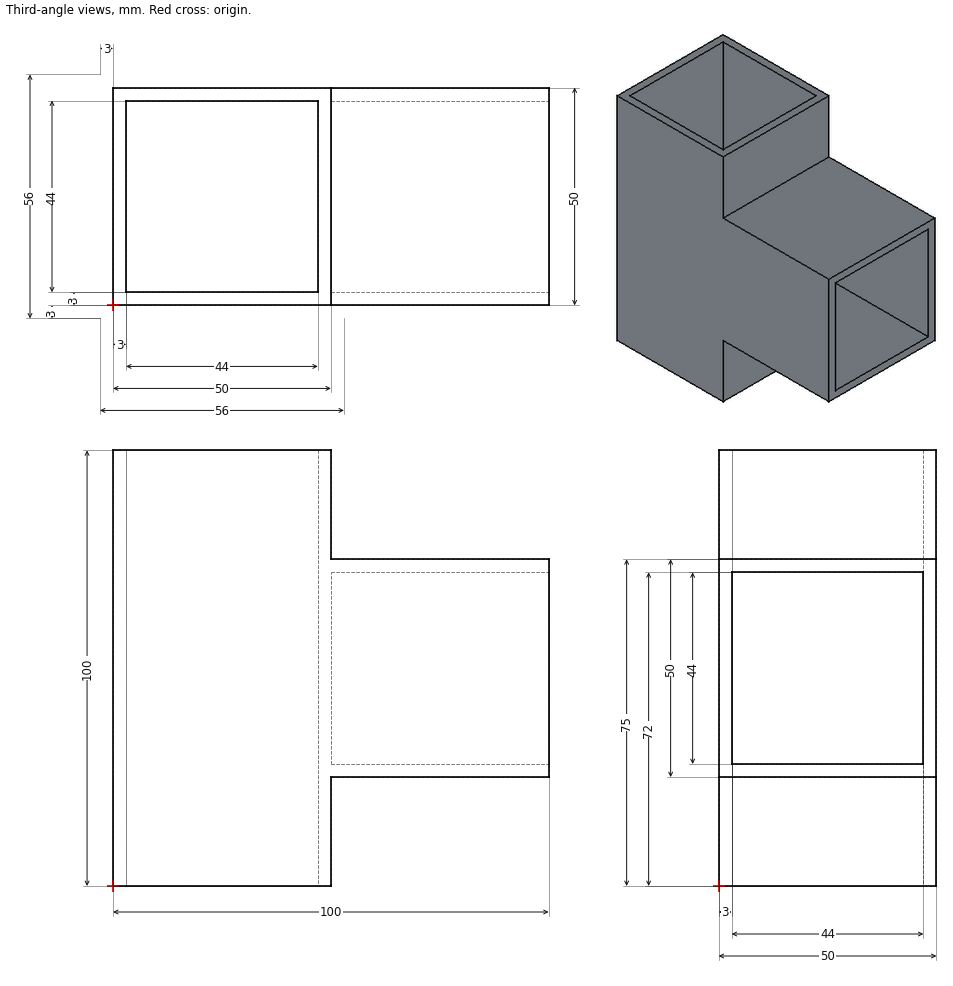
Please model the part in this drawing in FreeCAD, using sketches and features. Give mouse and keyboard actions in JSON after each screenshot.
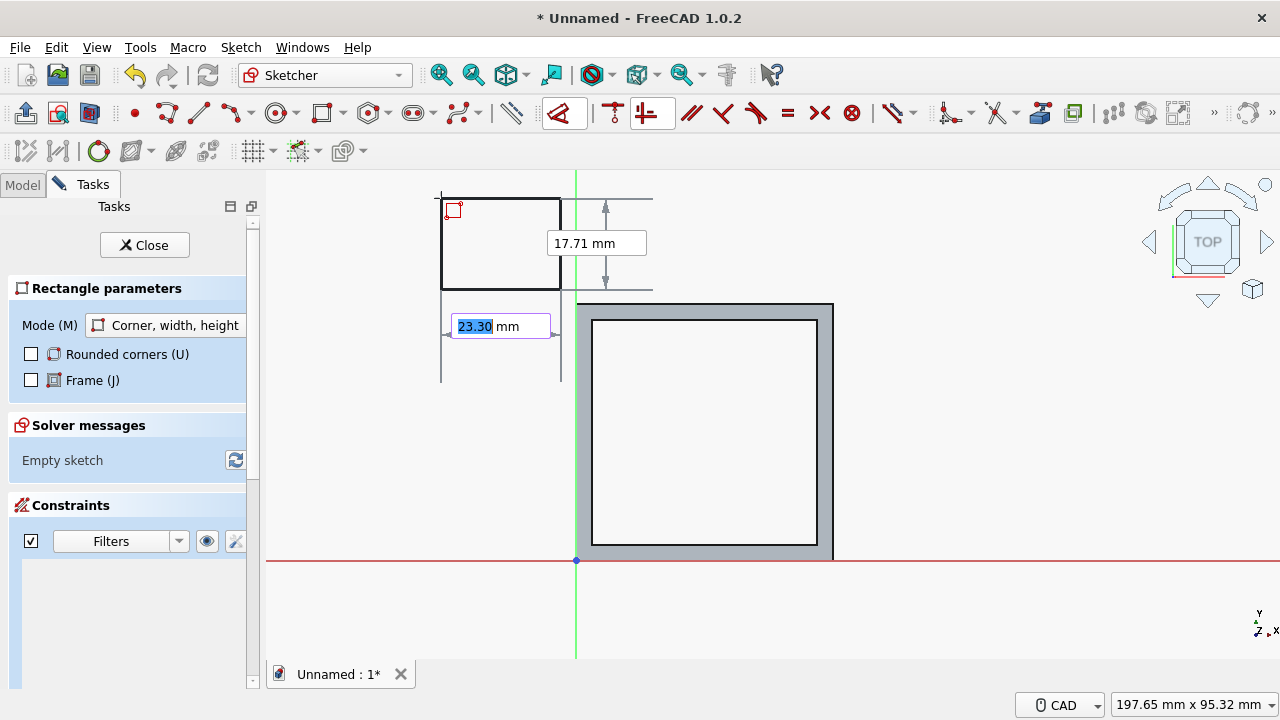
{"action": "left_click", "coordinate": [848, 576]}
{"action": "key", "text": "Escape"}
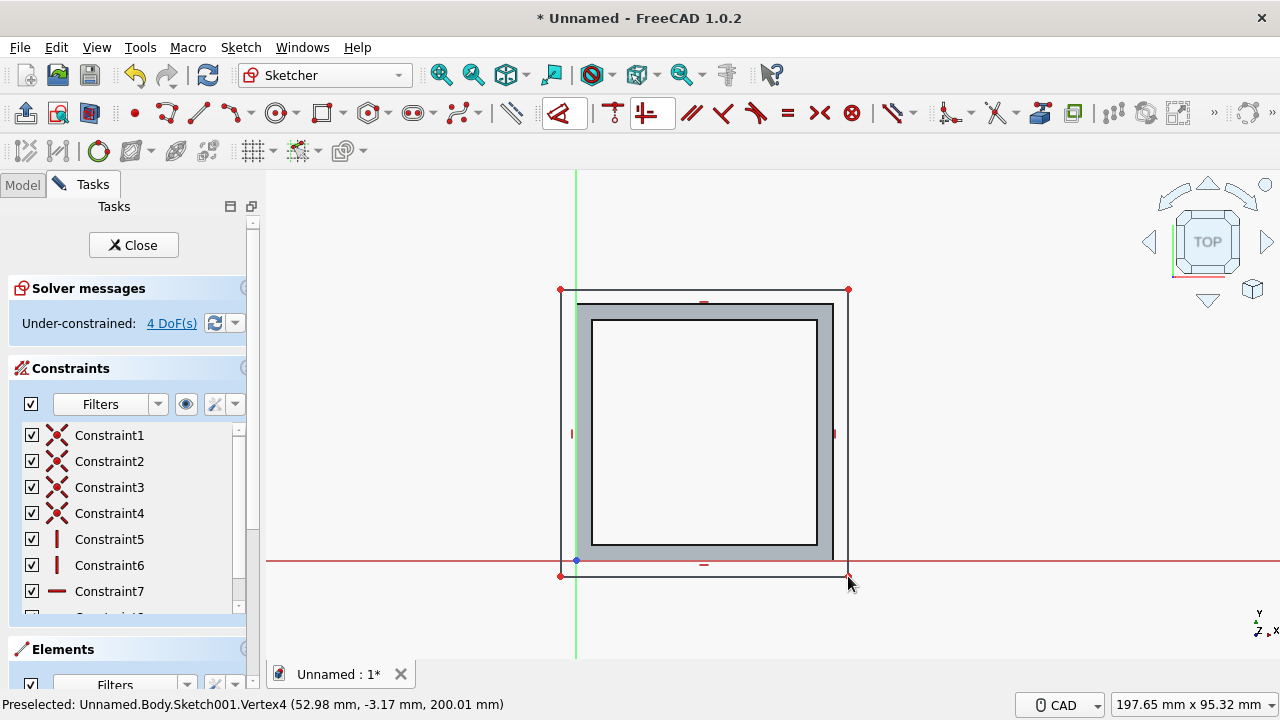
{"action": "left_click", "coordinate": [561, 376]}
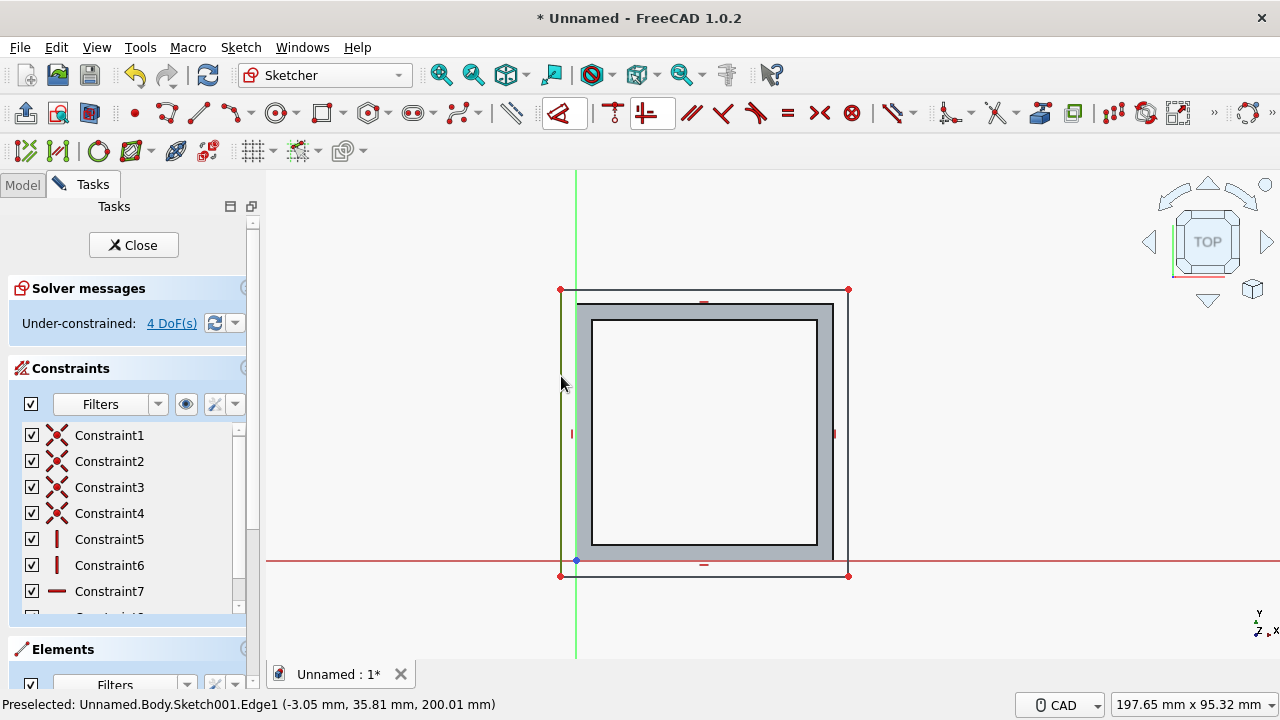
{"action": "key", "text": "i"}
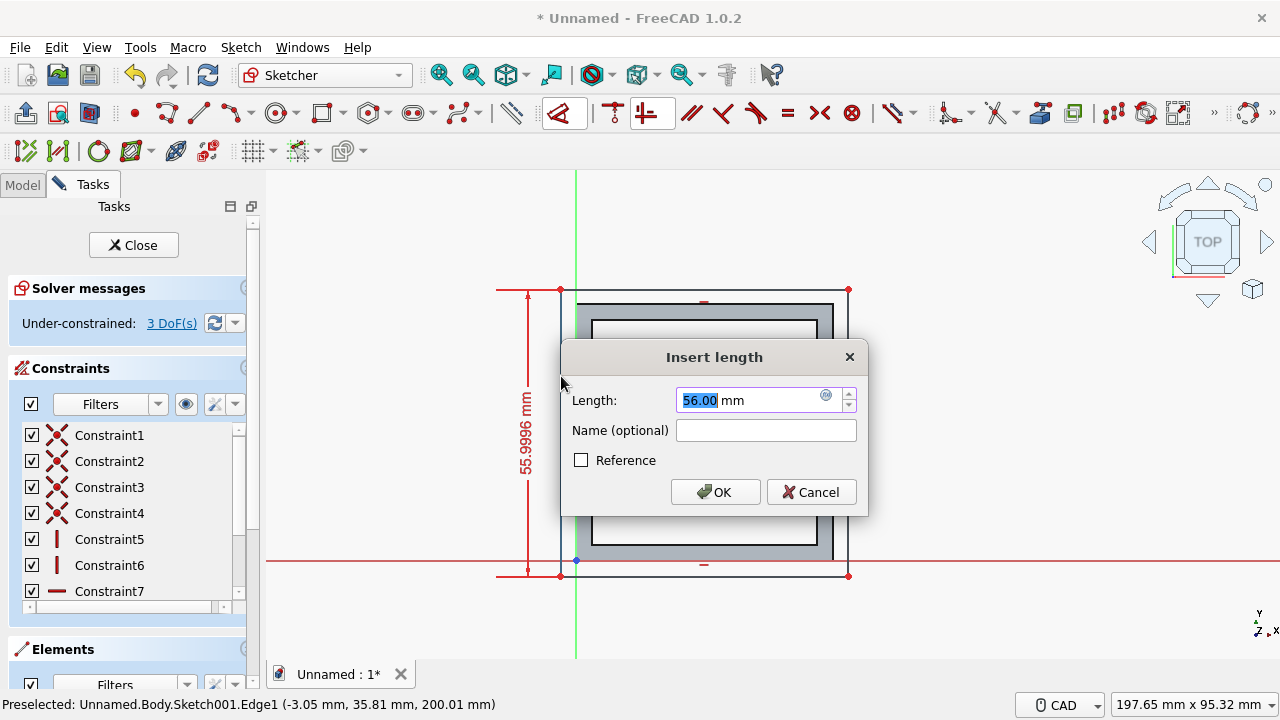
{"action": "type", "text": "56"}
{"action": "key", "text": "Return"}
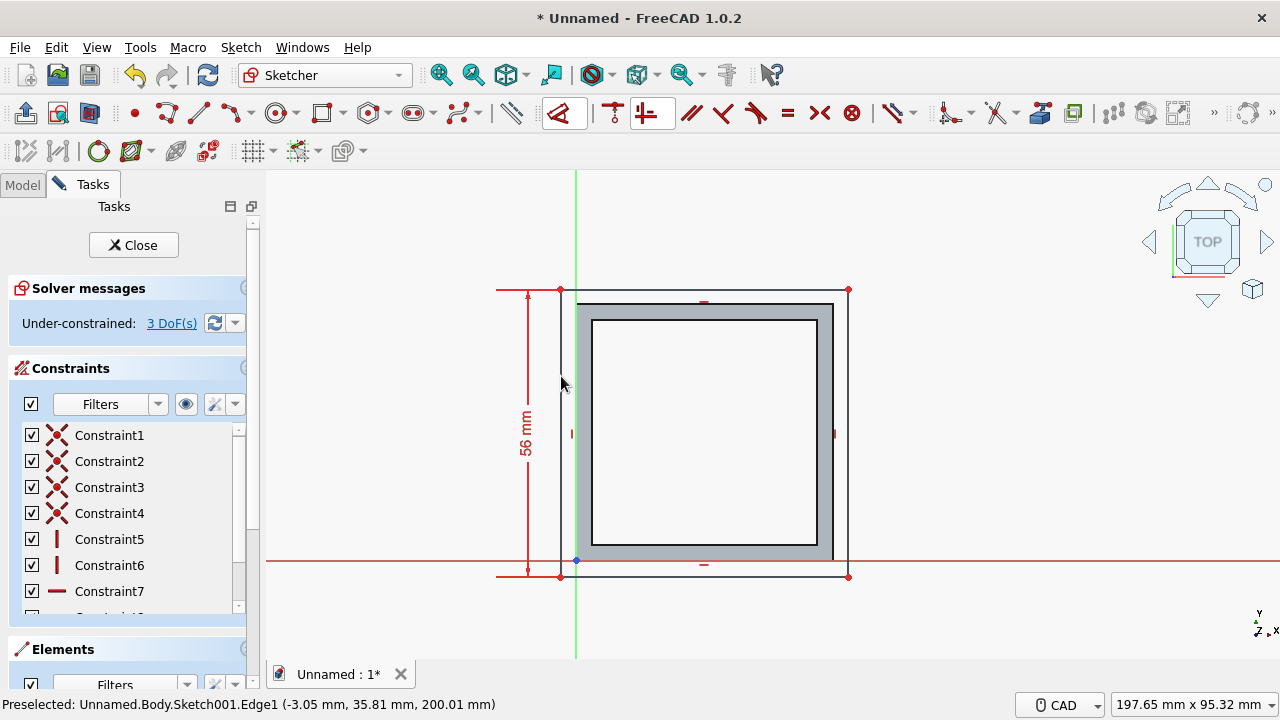
{"action": "left_click", "coordinate": [647, 577]}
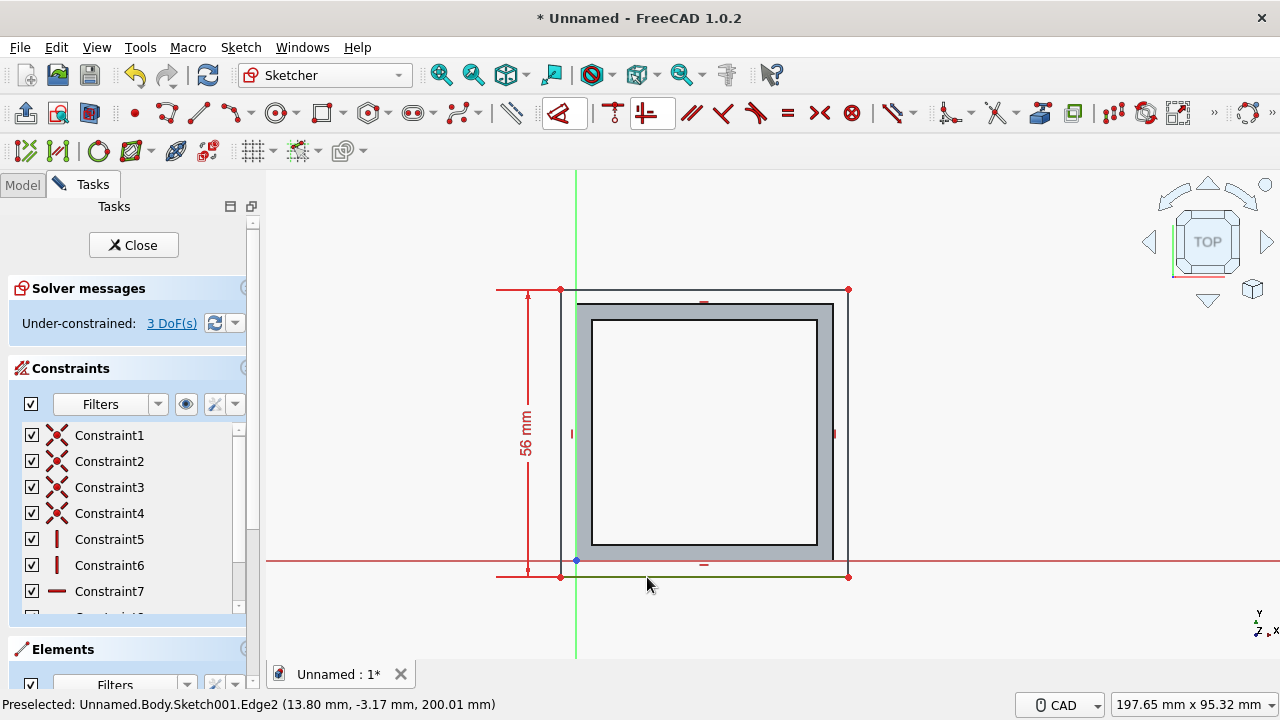
{"action": "key", "text": "l"}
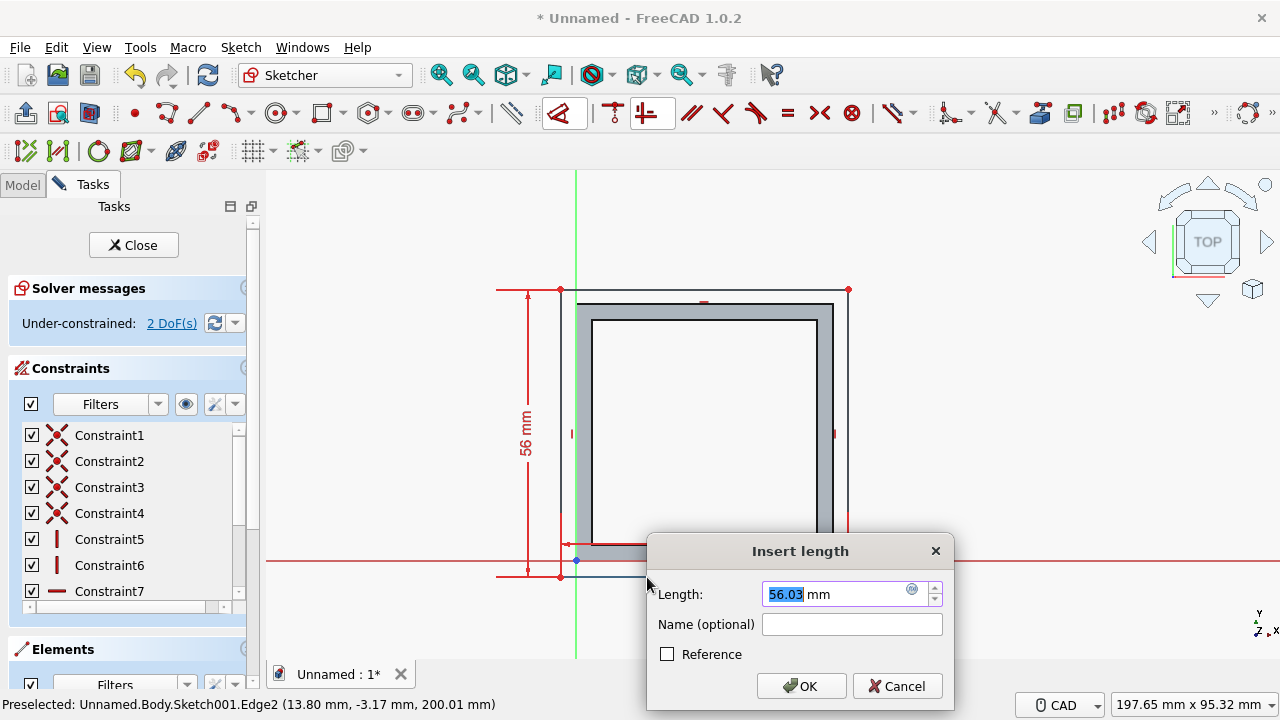
{"action": "type", "text": "56"}
{"action": "key", "text": "Return"}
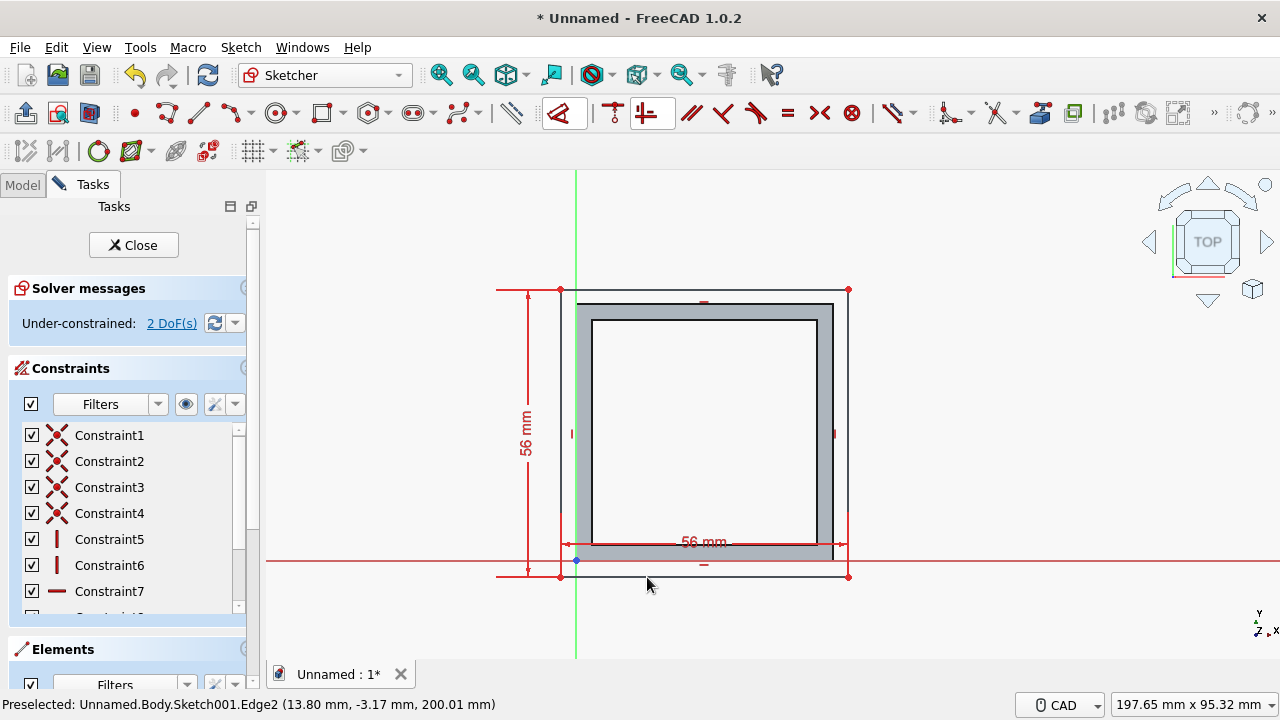
{"action": "scroll", "coordinate": [561, 290], "scroll_direction": "up", "scroll_amount": 5}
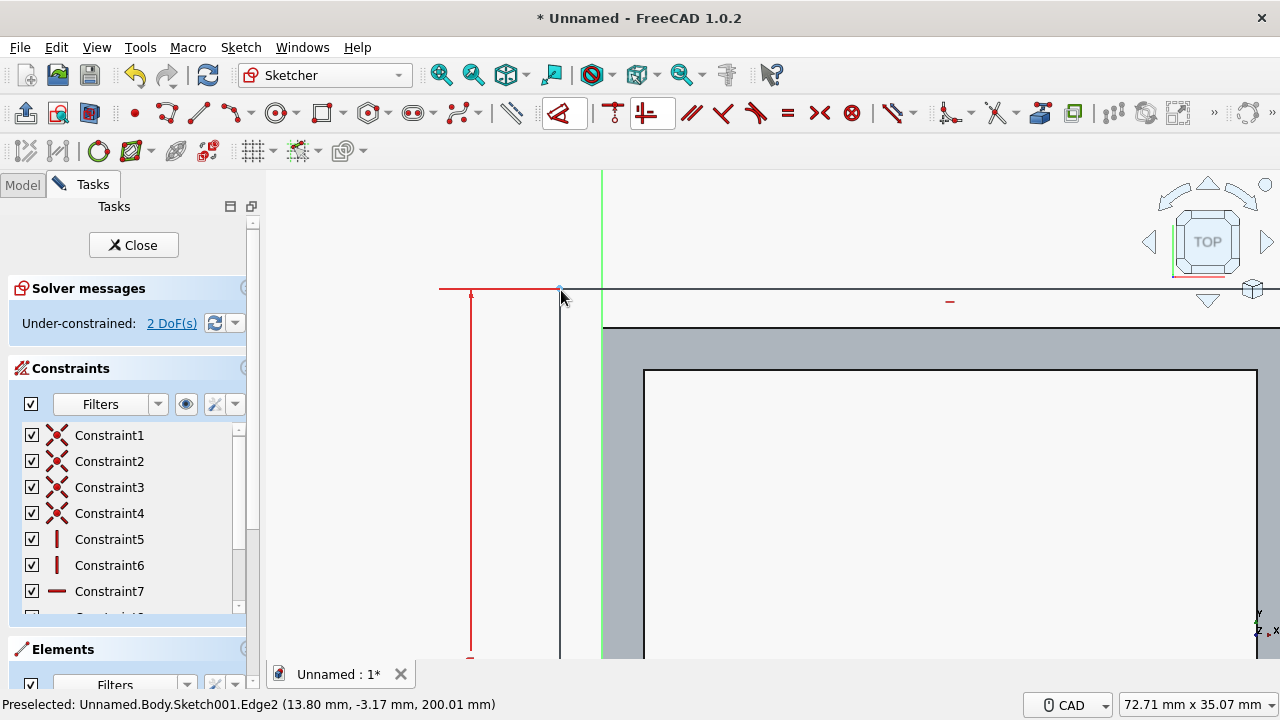
{"action": "left_click", "coordinate": [560, 289]}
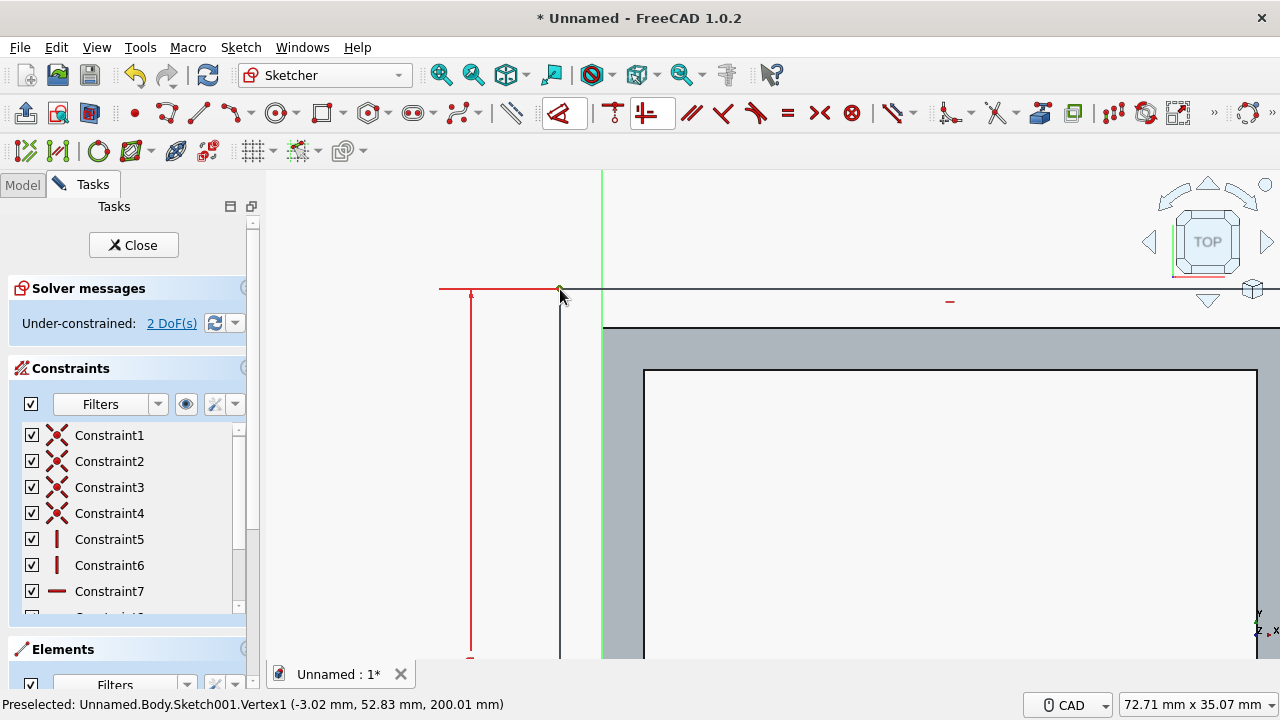
{"action": "key", "text": "l"}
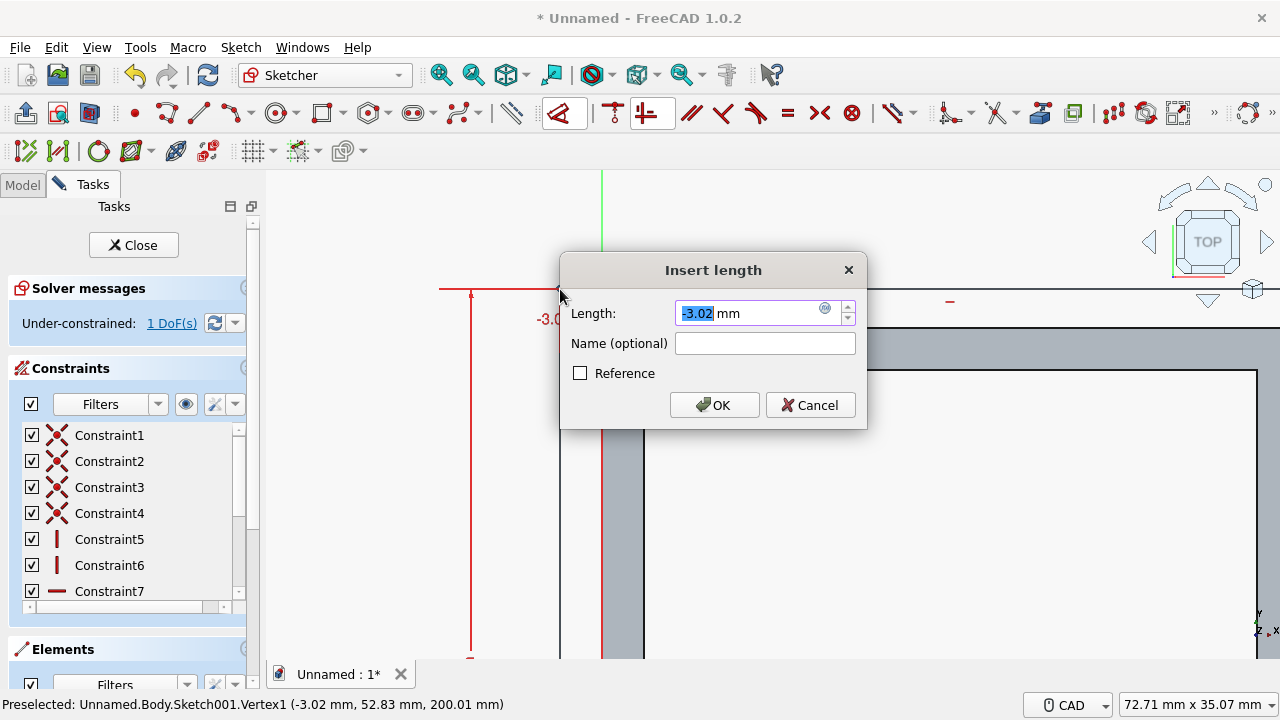
{"action": "type", "text": "-3"}
{"action": "key", "text": "Return"}